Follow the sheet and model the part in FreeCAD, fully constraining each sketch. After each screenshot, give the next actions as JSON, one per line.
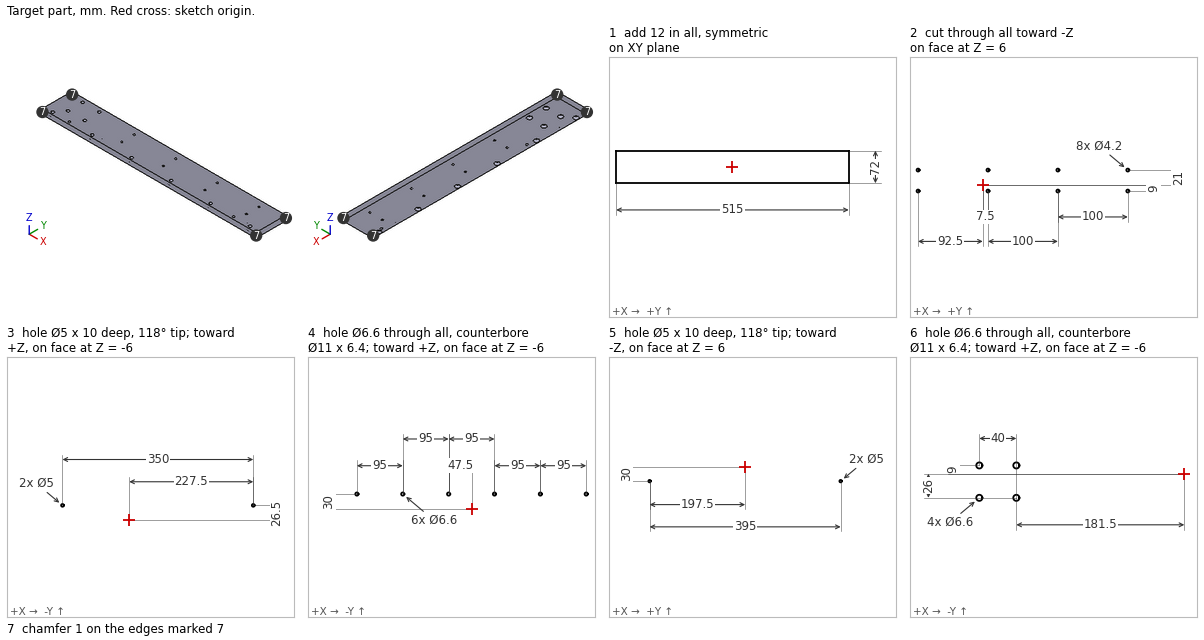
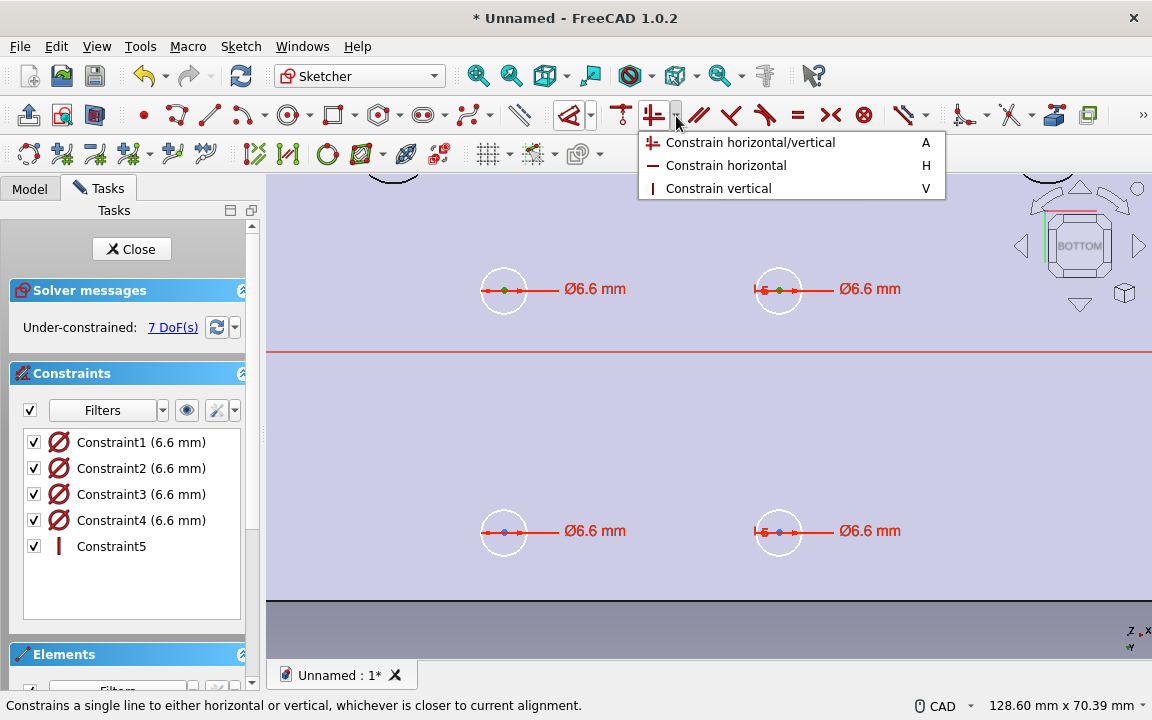
{"action": "left_click", "coordinate": [792, 166]}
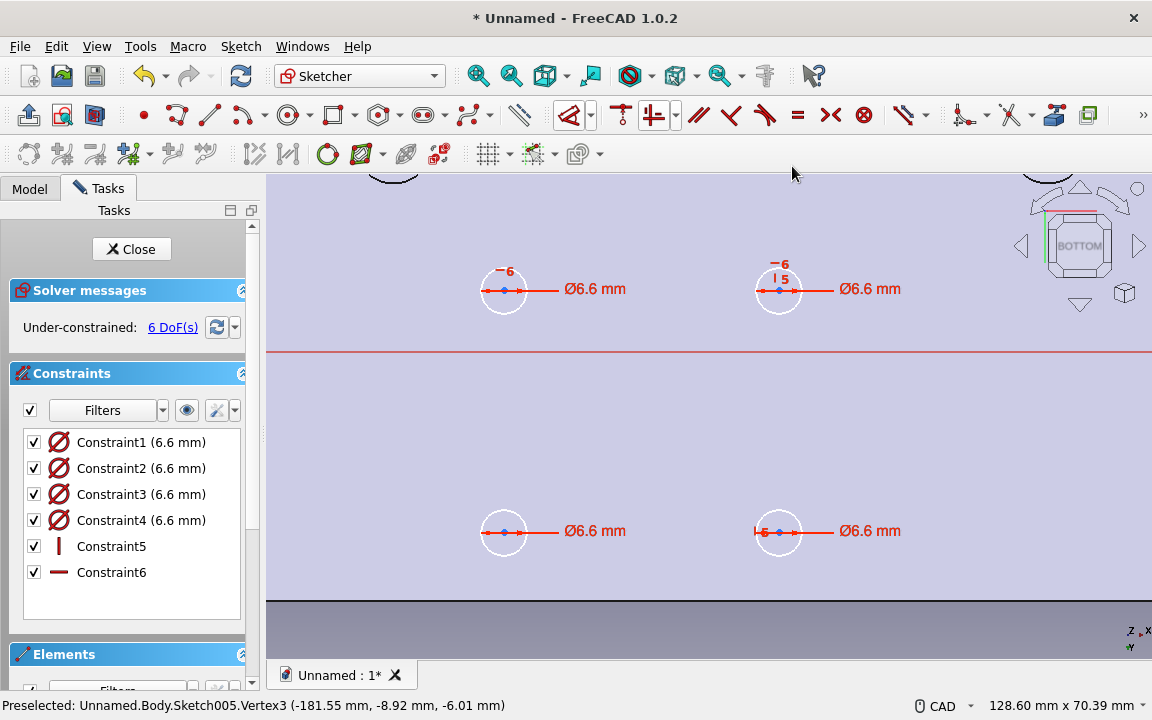
{"action": "left_click", "coordinate": [504, 291]}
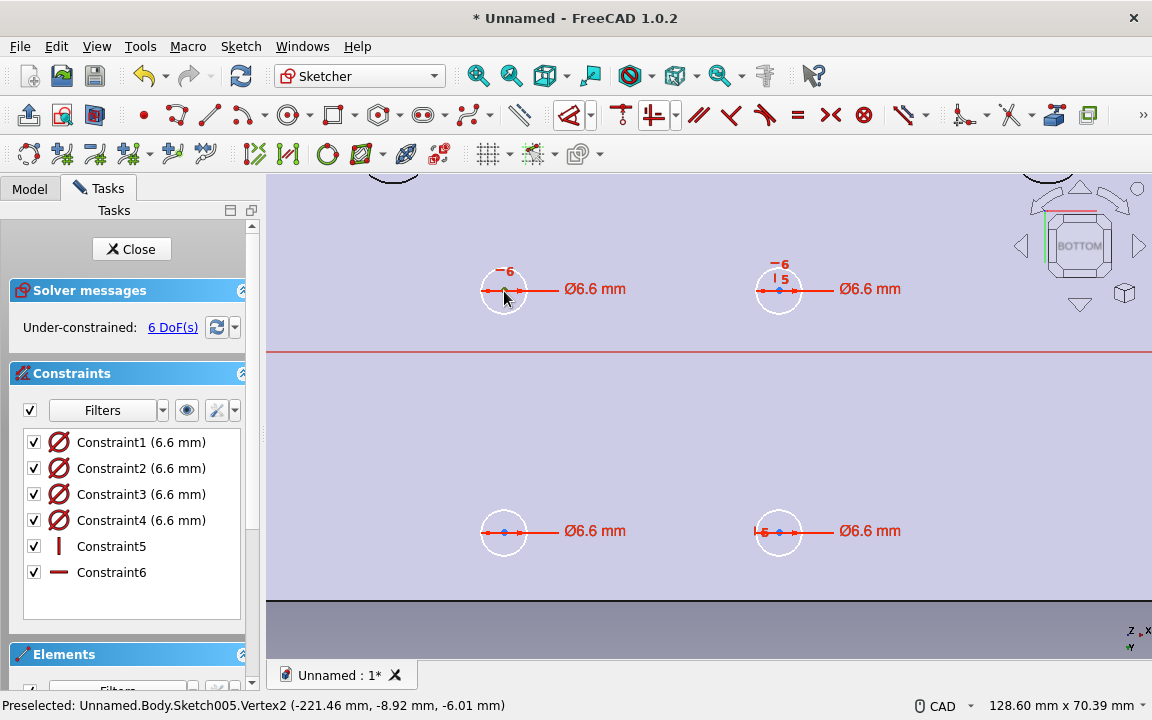
{"action": "left_click", "coordinate": [504, 533]}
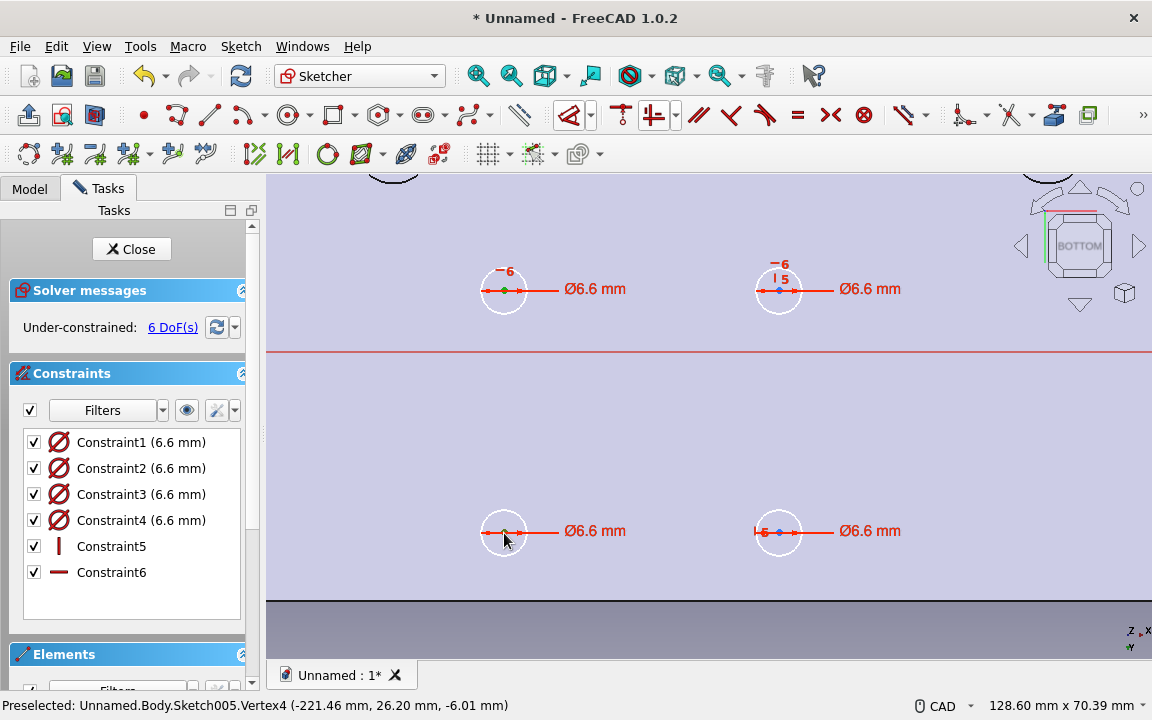
{"action": "left_click", "coordinate": [676, 116]}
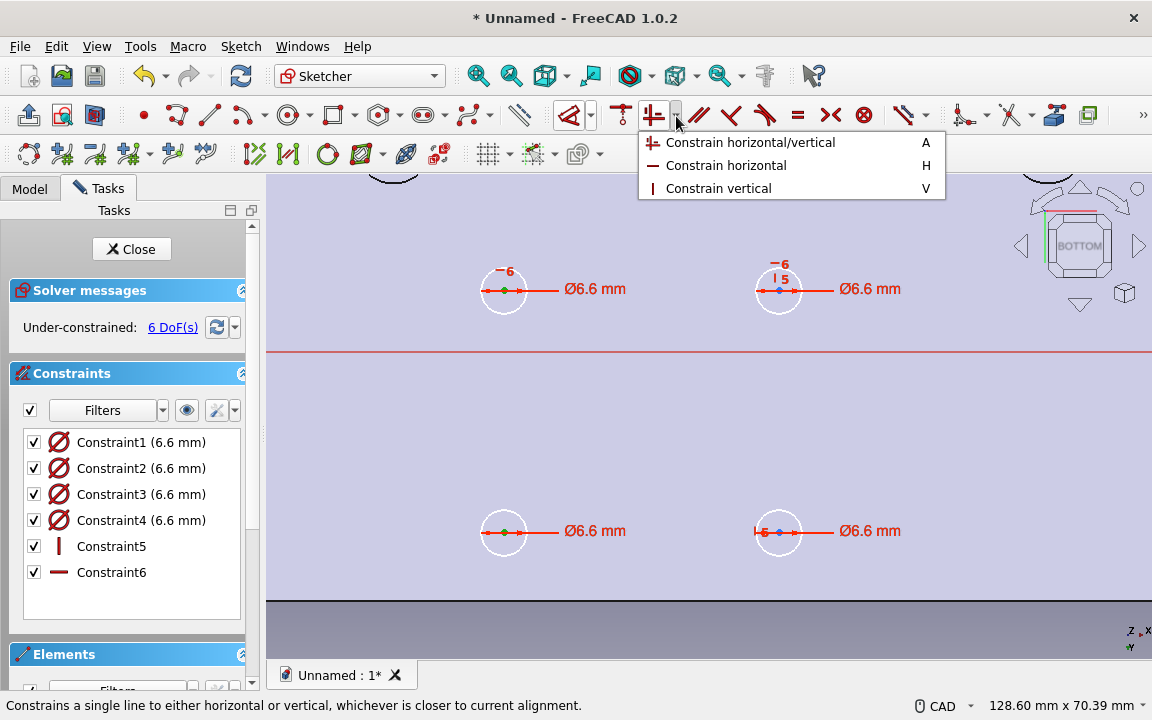
{"action": "left_click", "coordinate": [792, 188]}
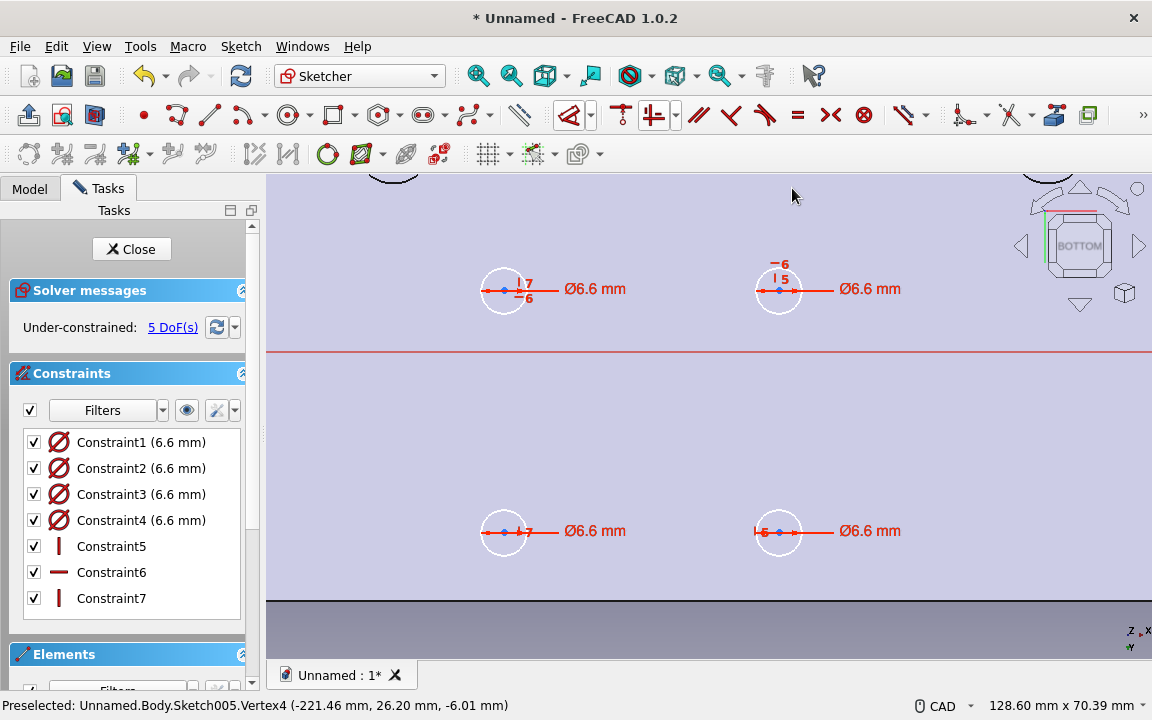
{"action": "left_click", "coordinate": [779, 533]}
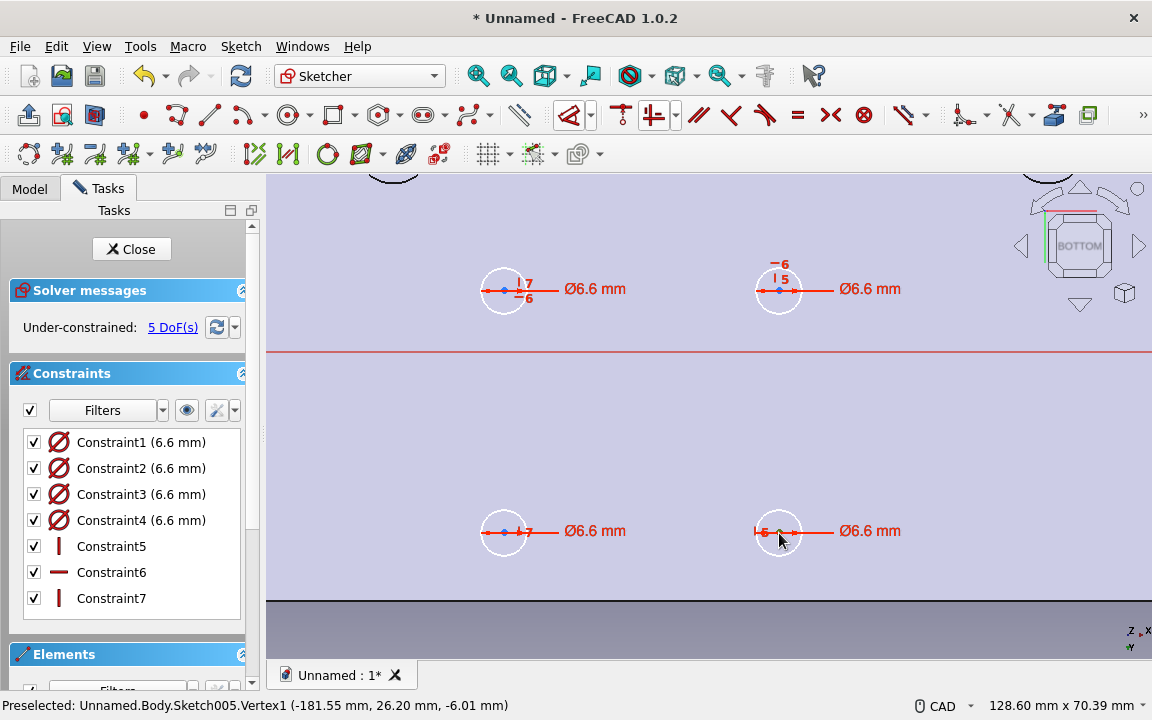
{"action": "left_click", "coordinate": [504, 533]}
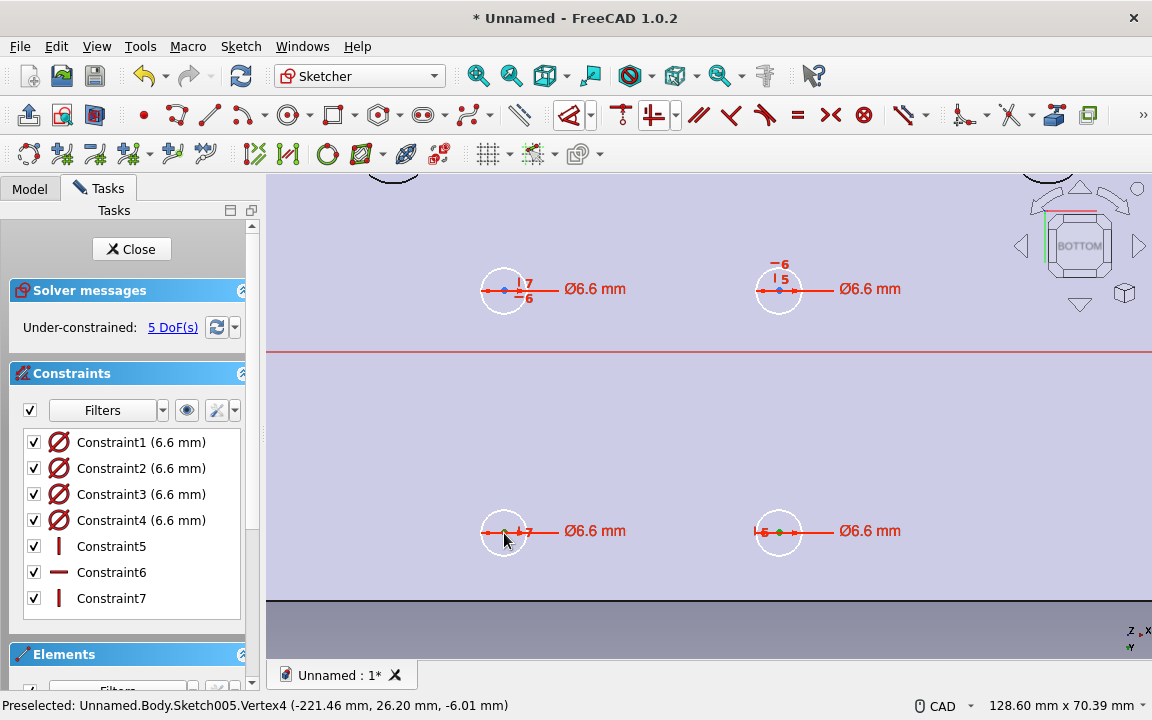
{"action": "key", "text": "h"}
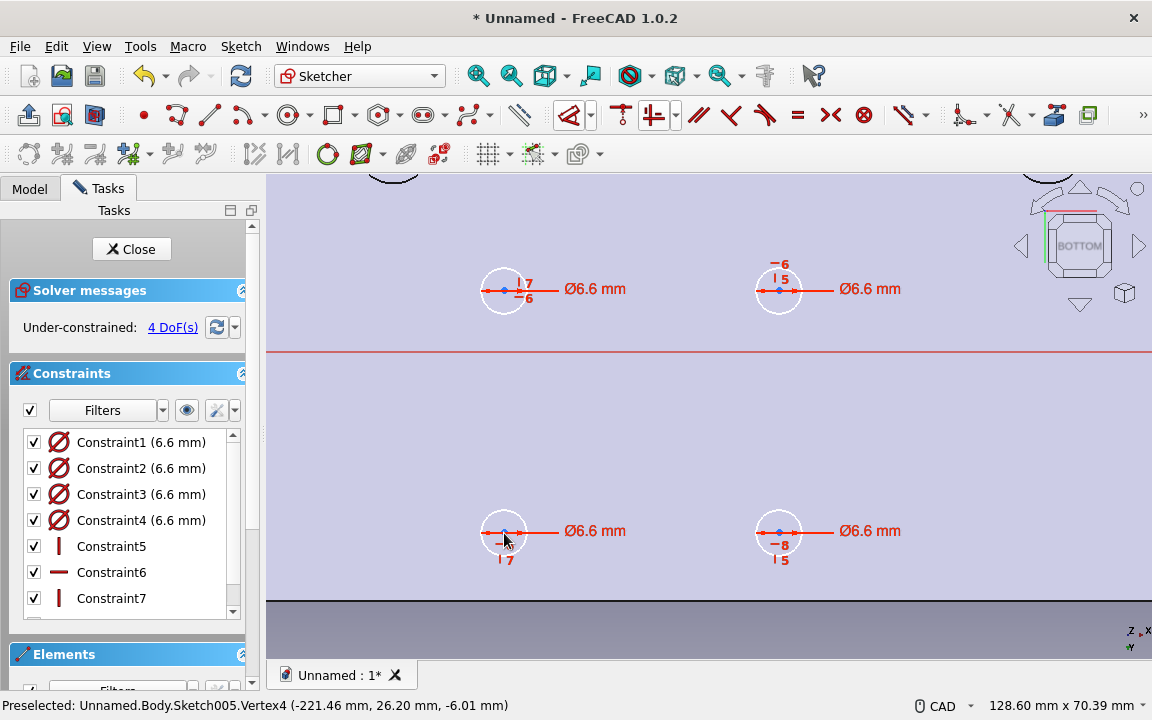
{"action": "left_click", "coordinate": [504, 291]}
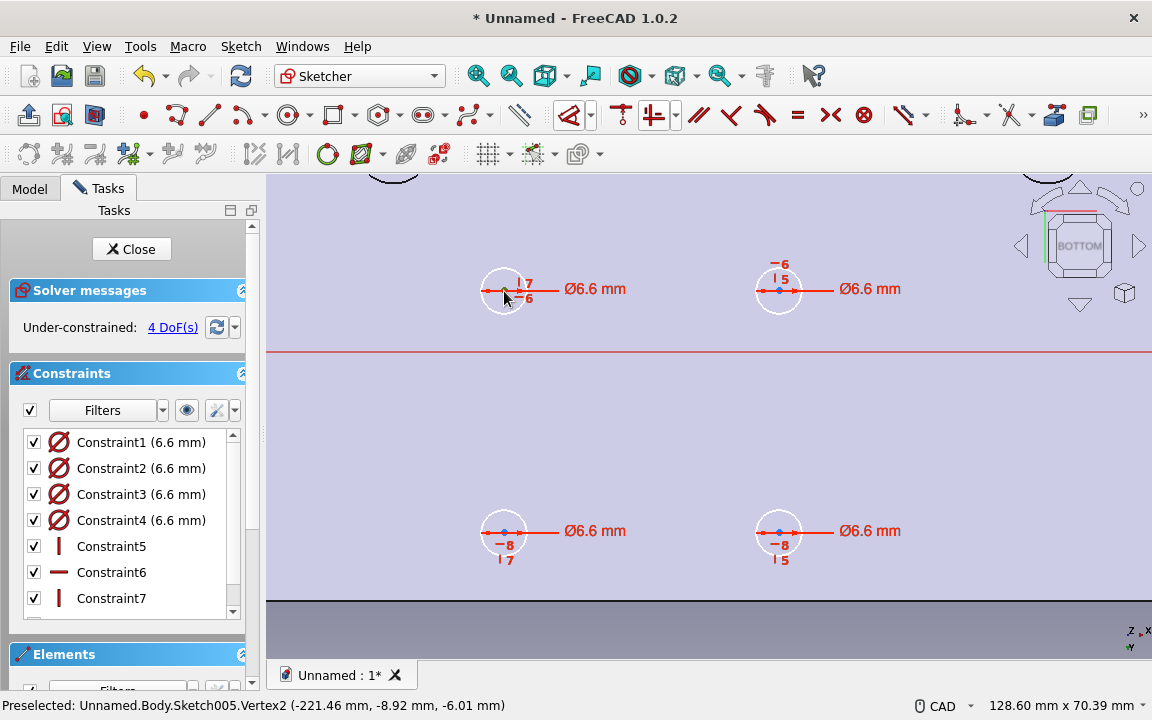
{"action": "left_click", "coordinate": [590, 116]}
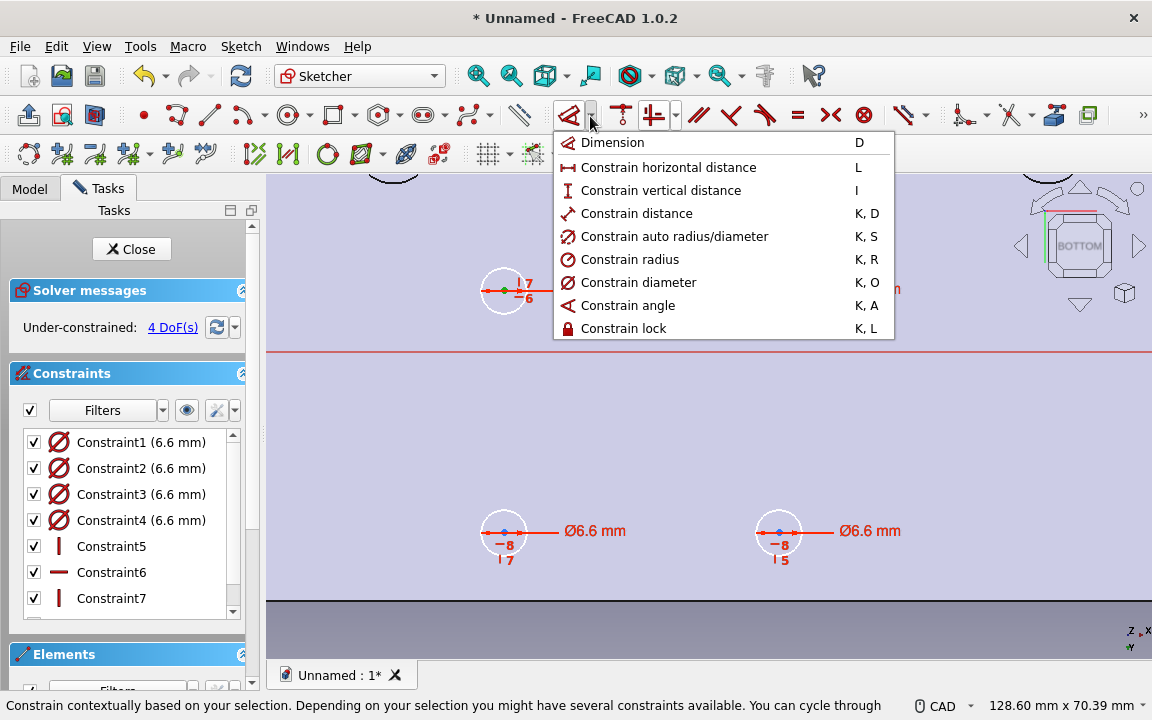
{"action": "left_click", "coordinate": [724, 190]}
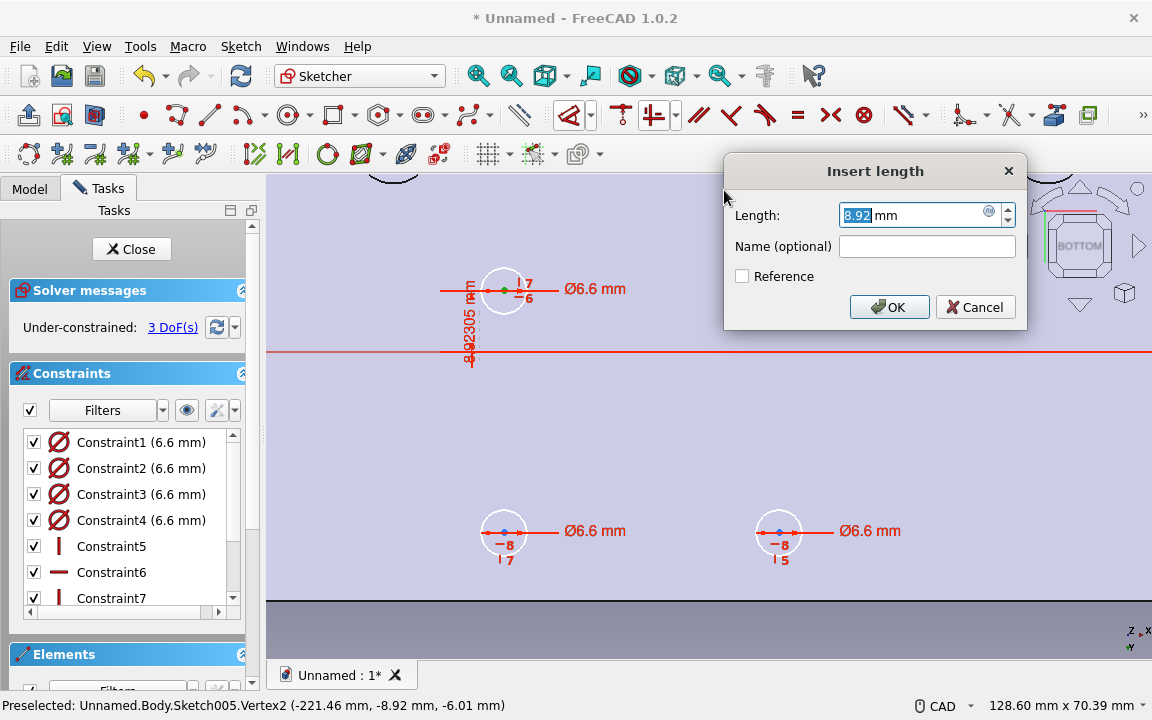
{"action": "type", "text": "9"}
{"action": "key", "text": "Return"}